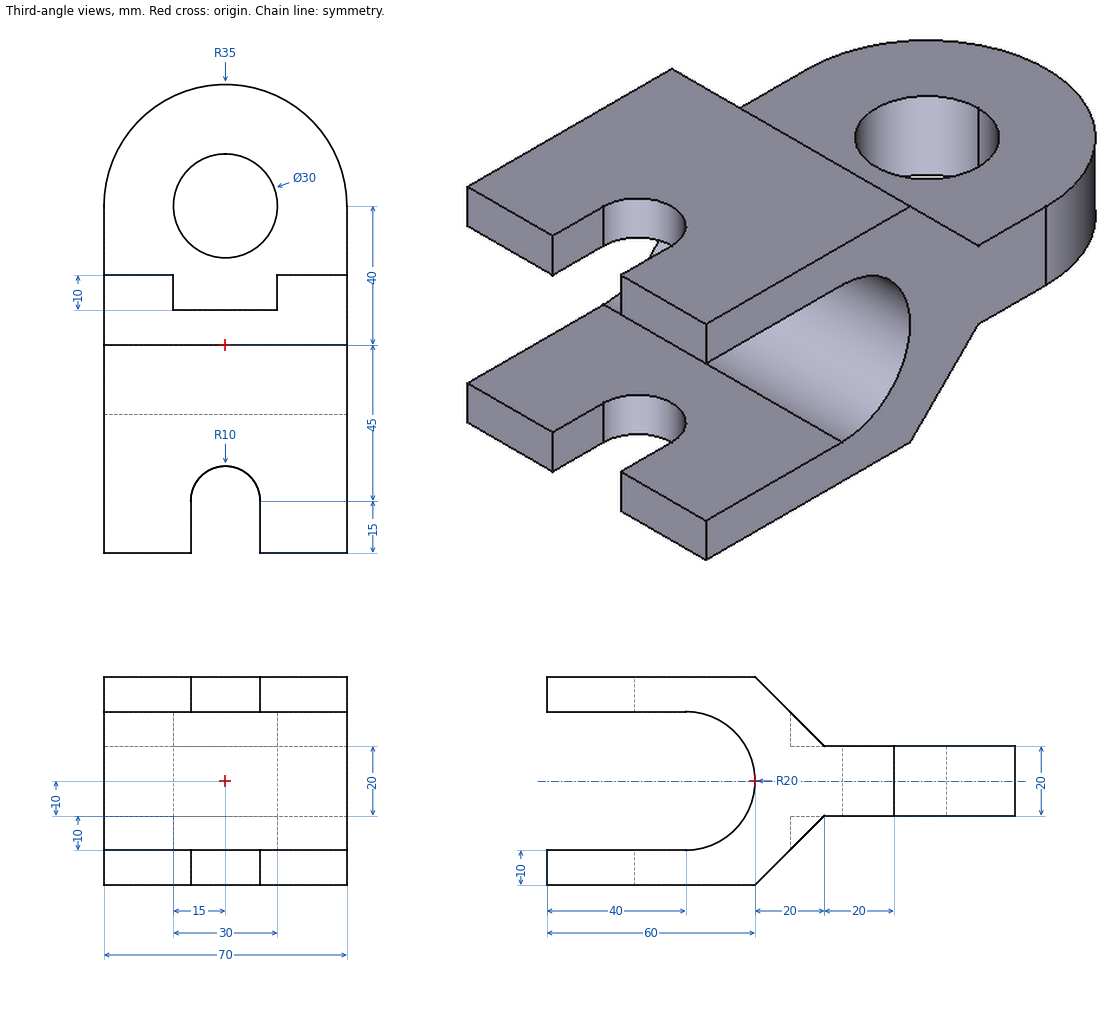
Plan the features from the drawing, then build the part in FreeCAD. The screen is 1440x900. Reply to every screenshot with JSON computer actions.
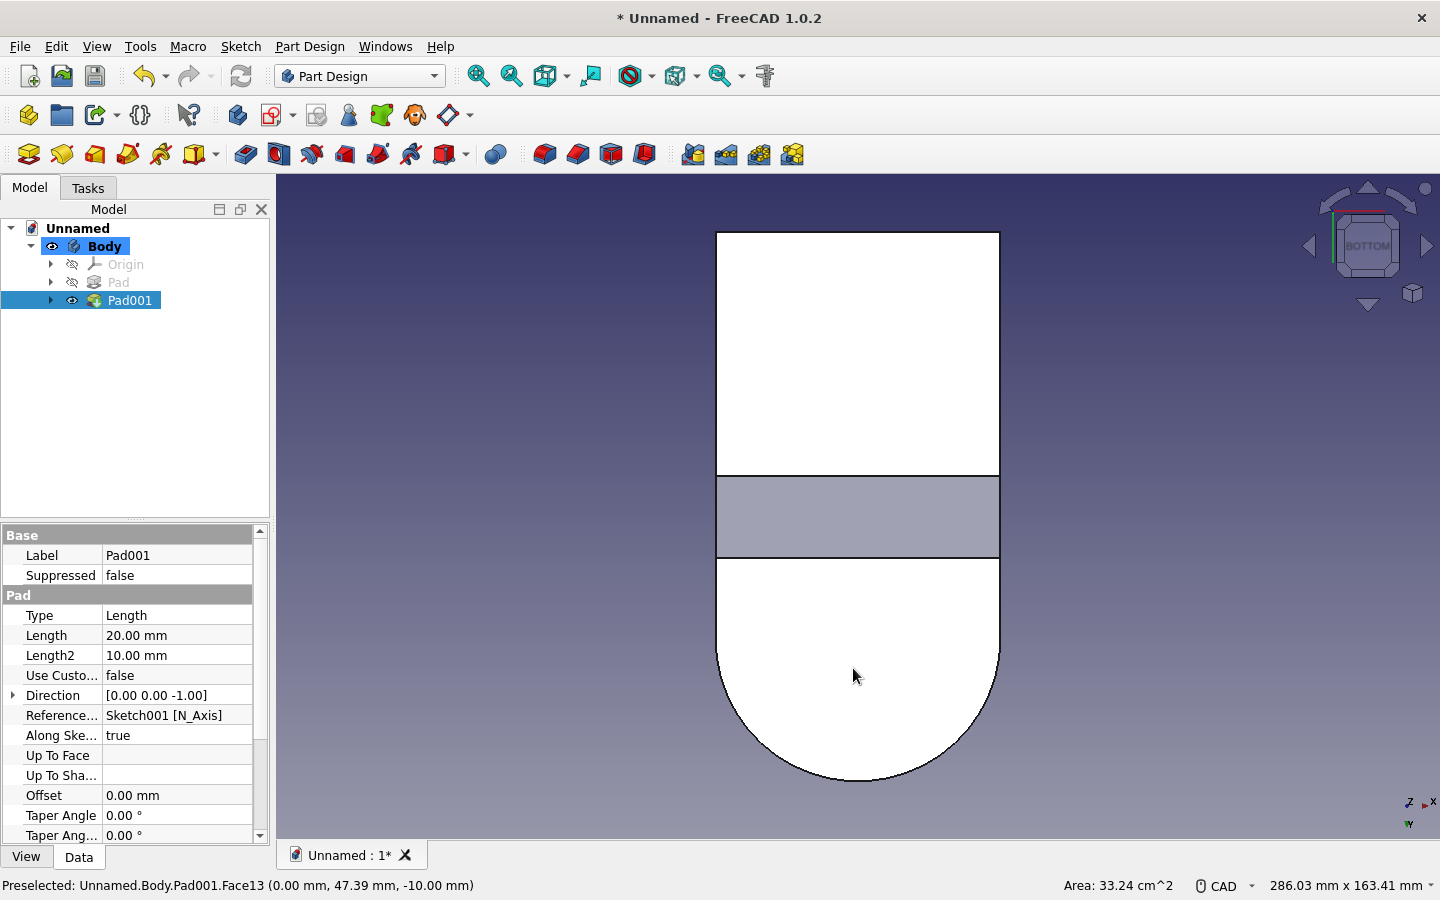
{"action": "left_click", "coordinate": [270, 116]}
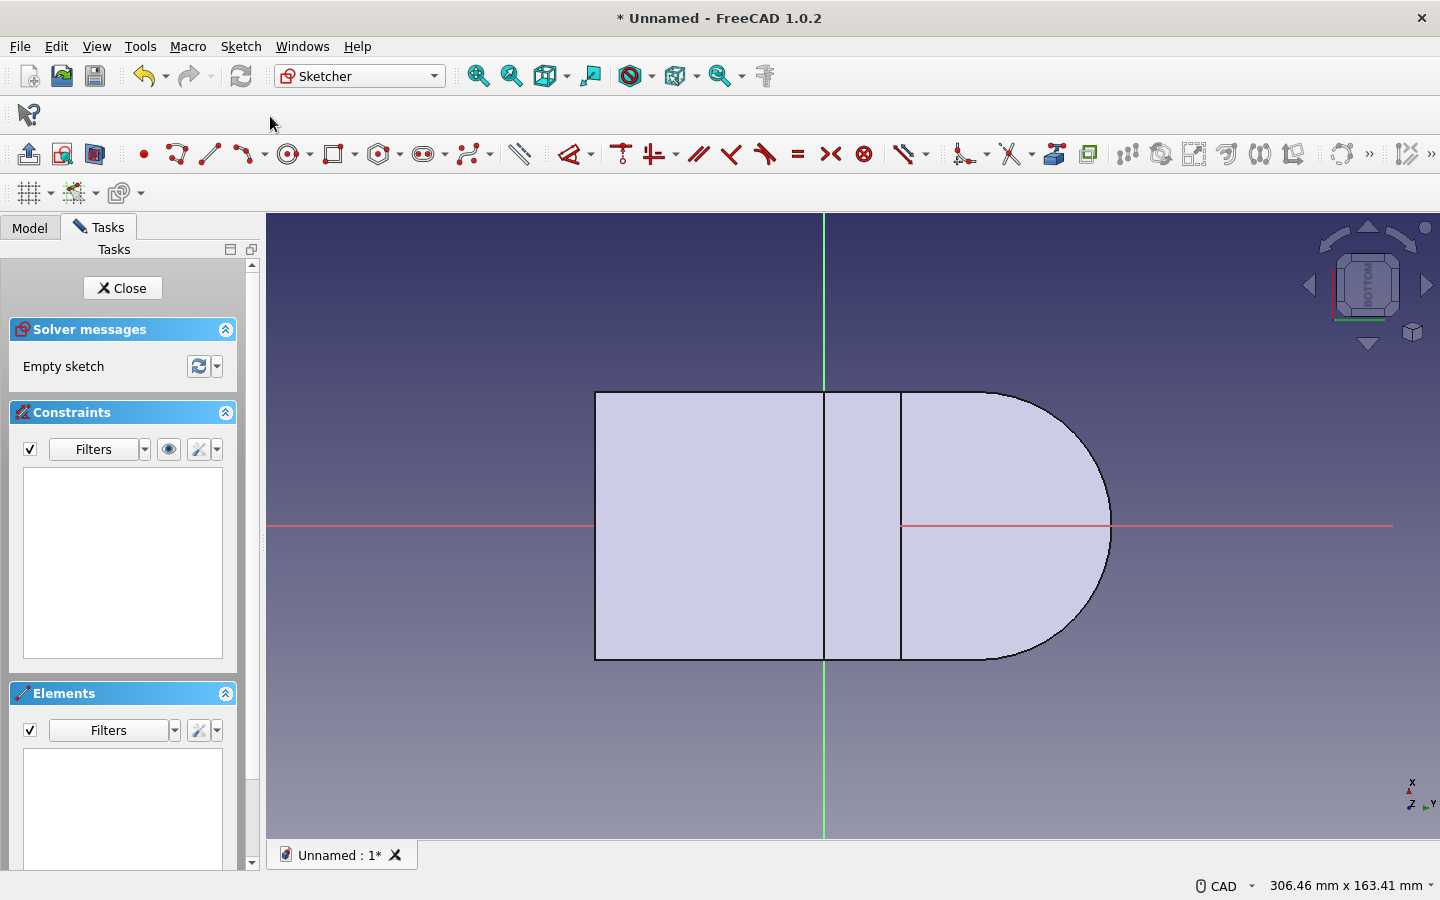
{"action": "key", "text": "q s"}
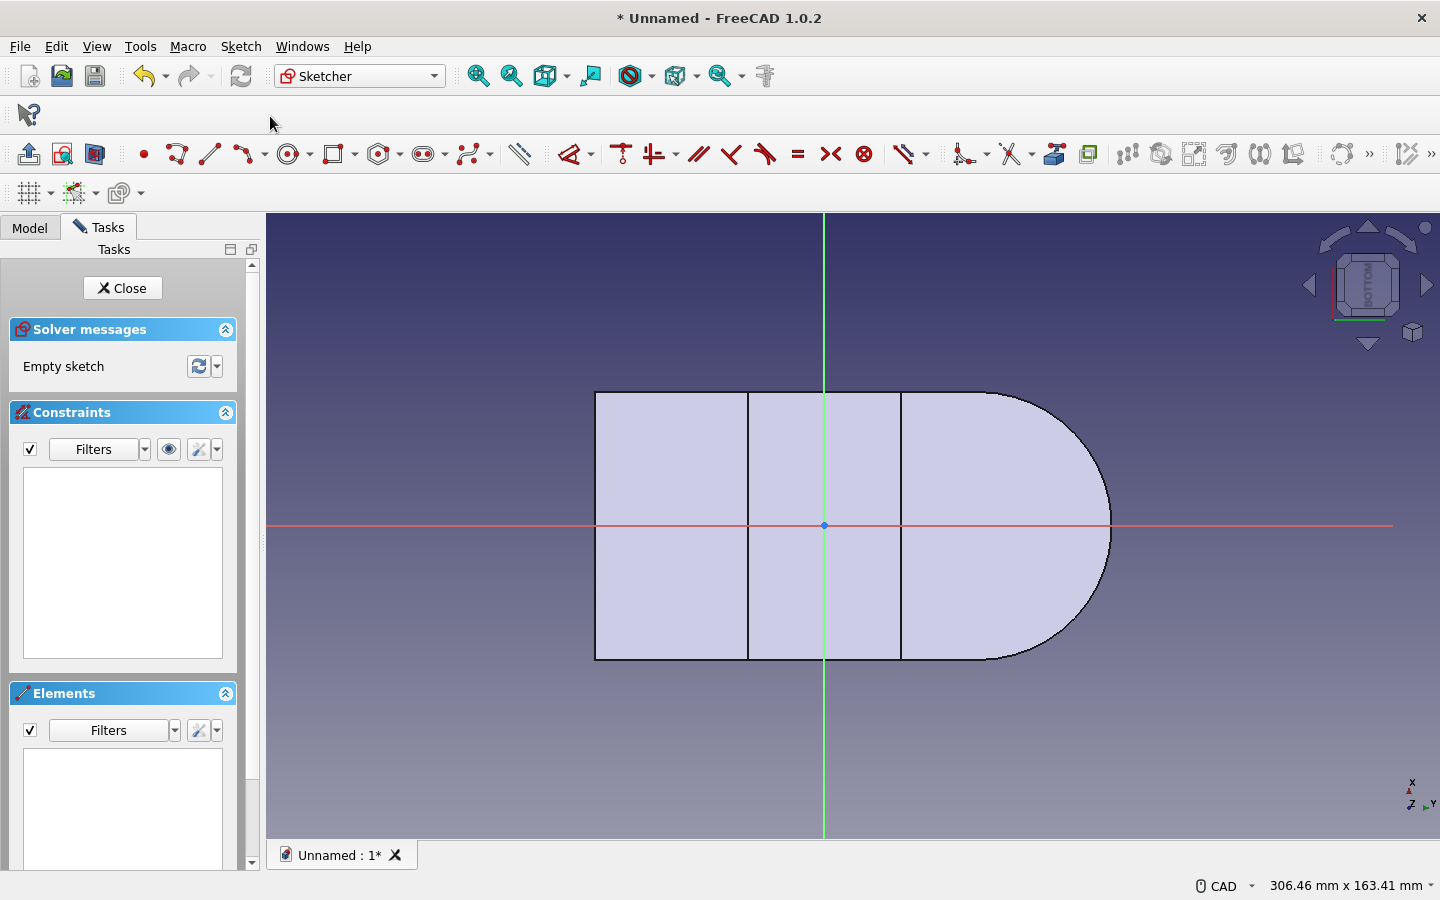
{"action": "scroll", "coordinate": [877, 526], "scroll_direction": "up", "scroll_amount": 2}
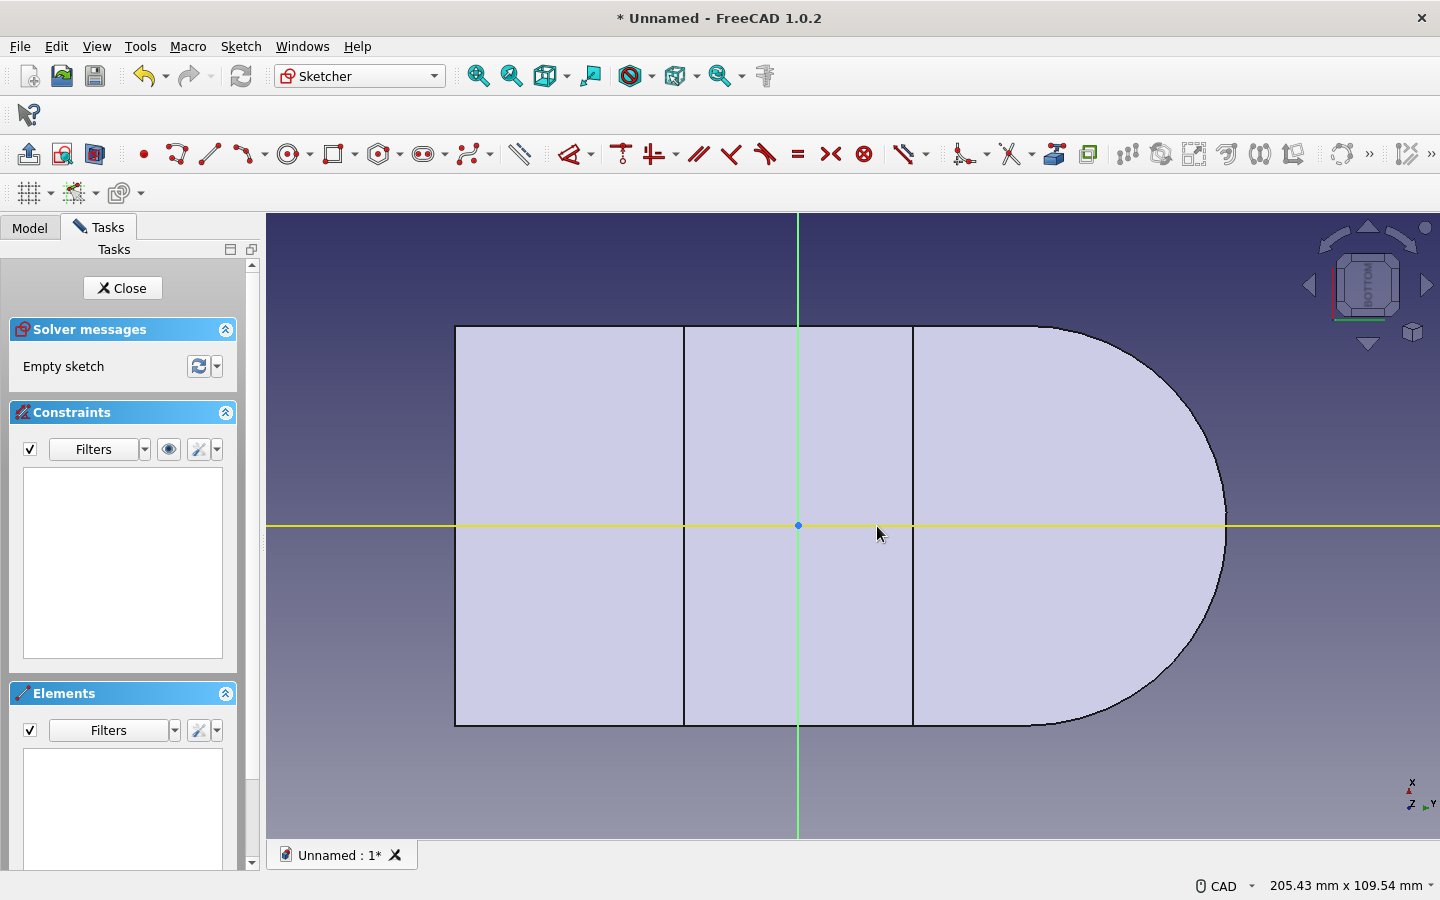
{"action": "left_click", "coordinate": [177, 154]}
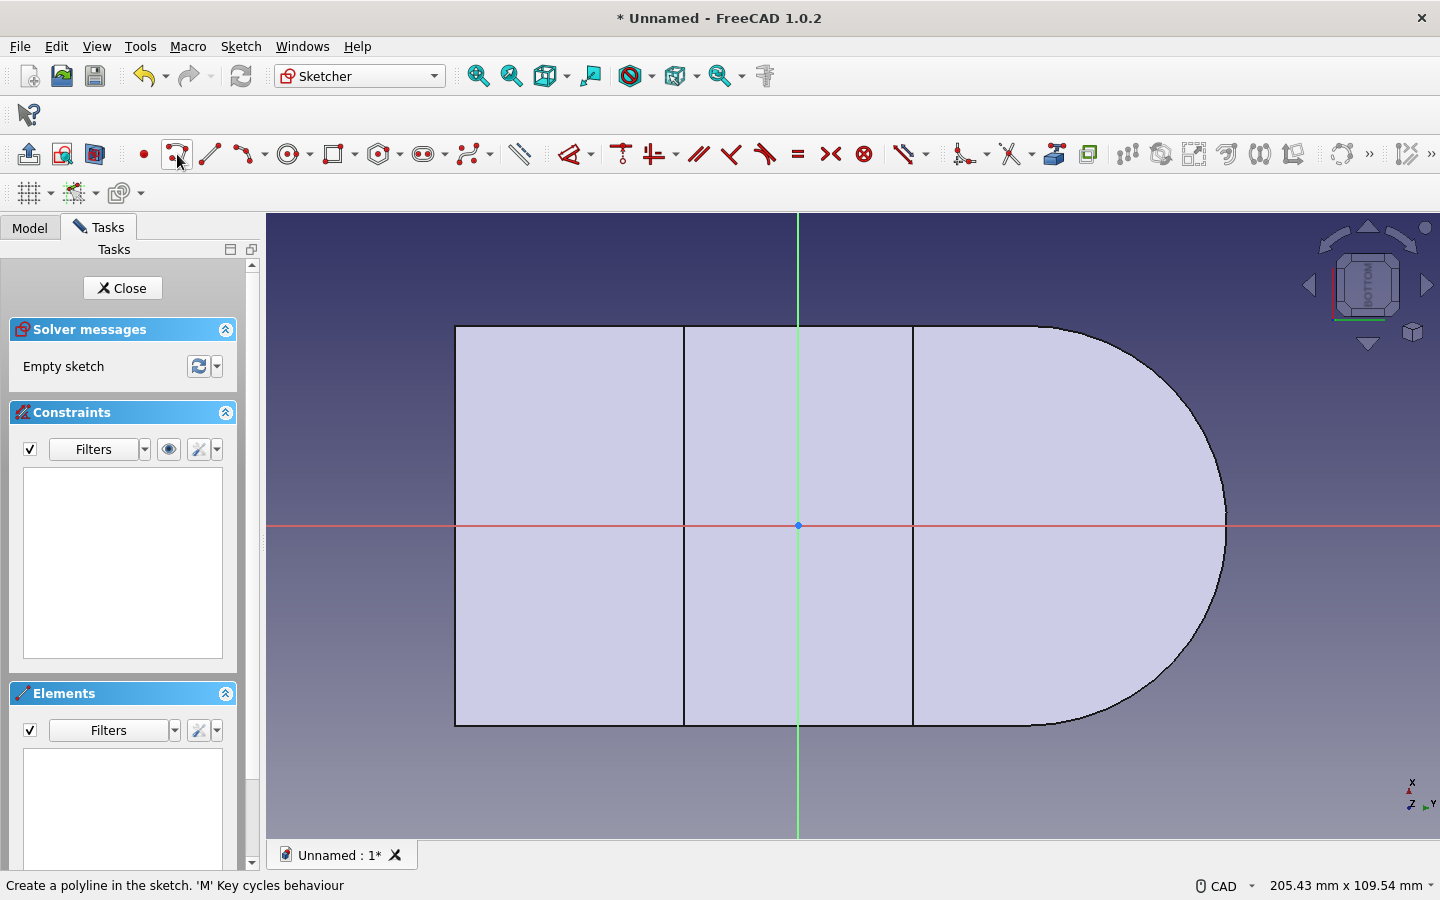
{"action": "left_click", "coordinate": [541, 469]}
{"action": "left_click", "coordinate": [455, 469]}
{"action": "left_click", "coordinate": [455, 583]}
{"action": "left_click", "coordinate": [541, 583]}
{"action": "right_click", "coordinate": [541, 583]}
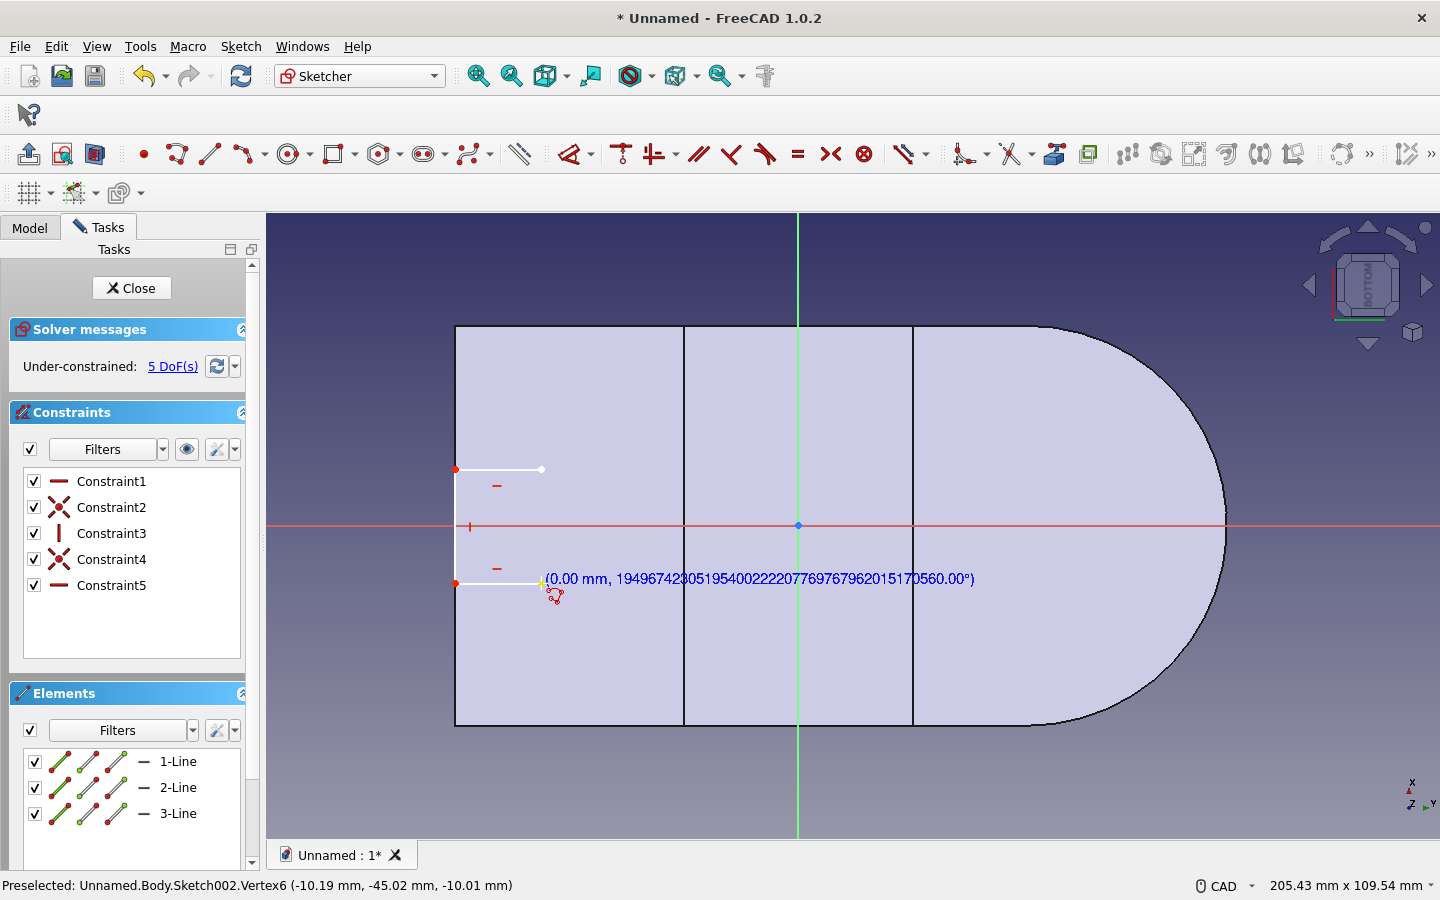
{"action": "key", "text": "g 3 a"}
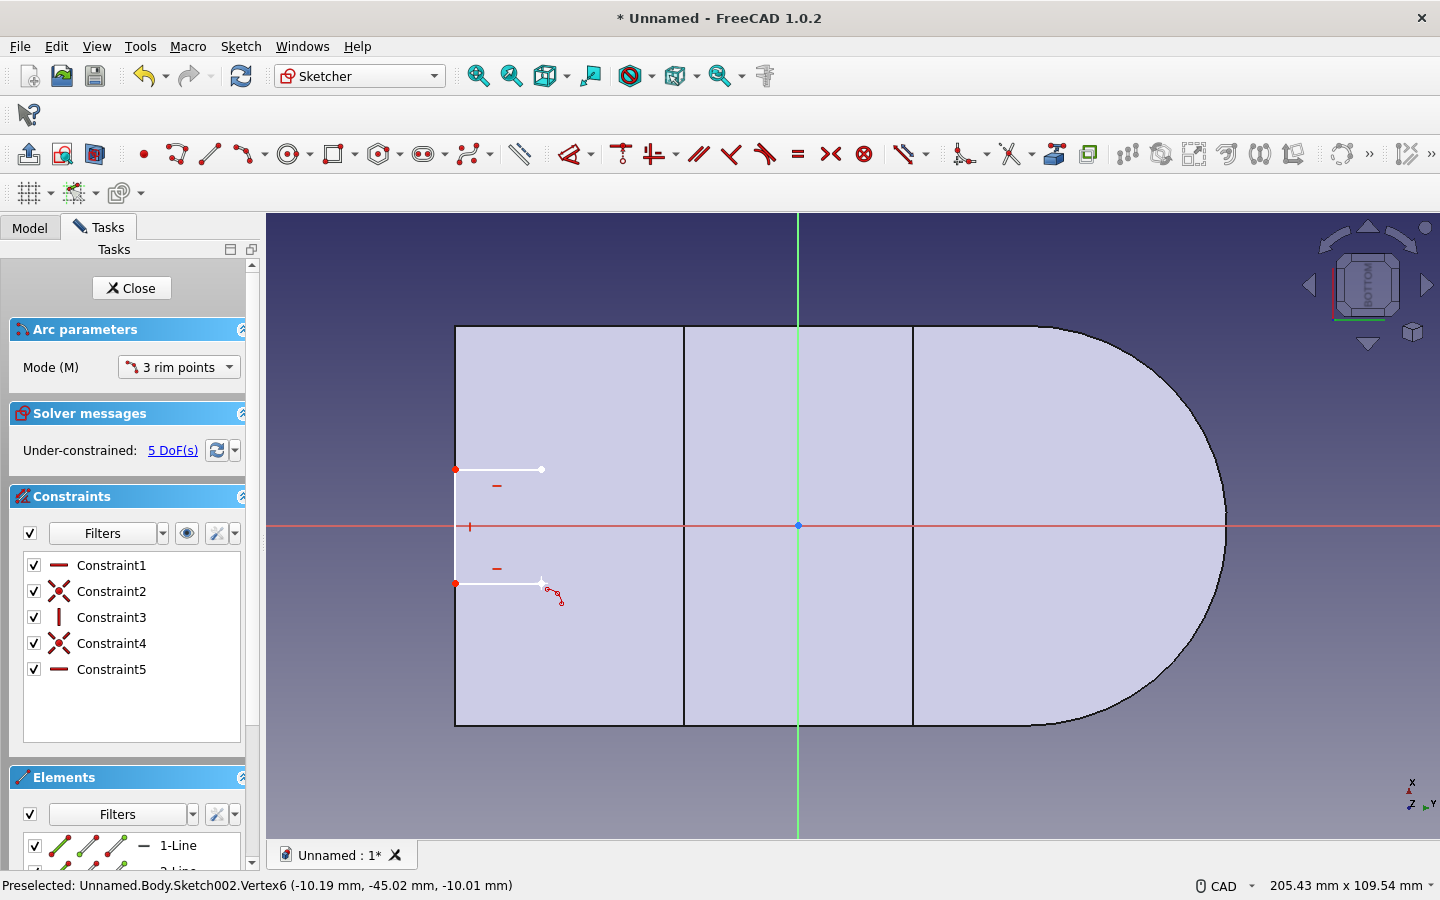
{"action": "left_click", "coordinate": [541, 584]}
{"action": "left_click", "coordinate": [541, 470]}
{"action": "left_click", "coordinate": [595, 543]}